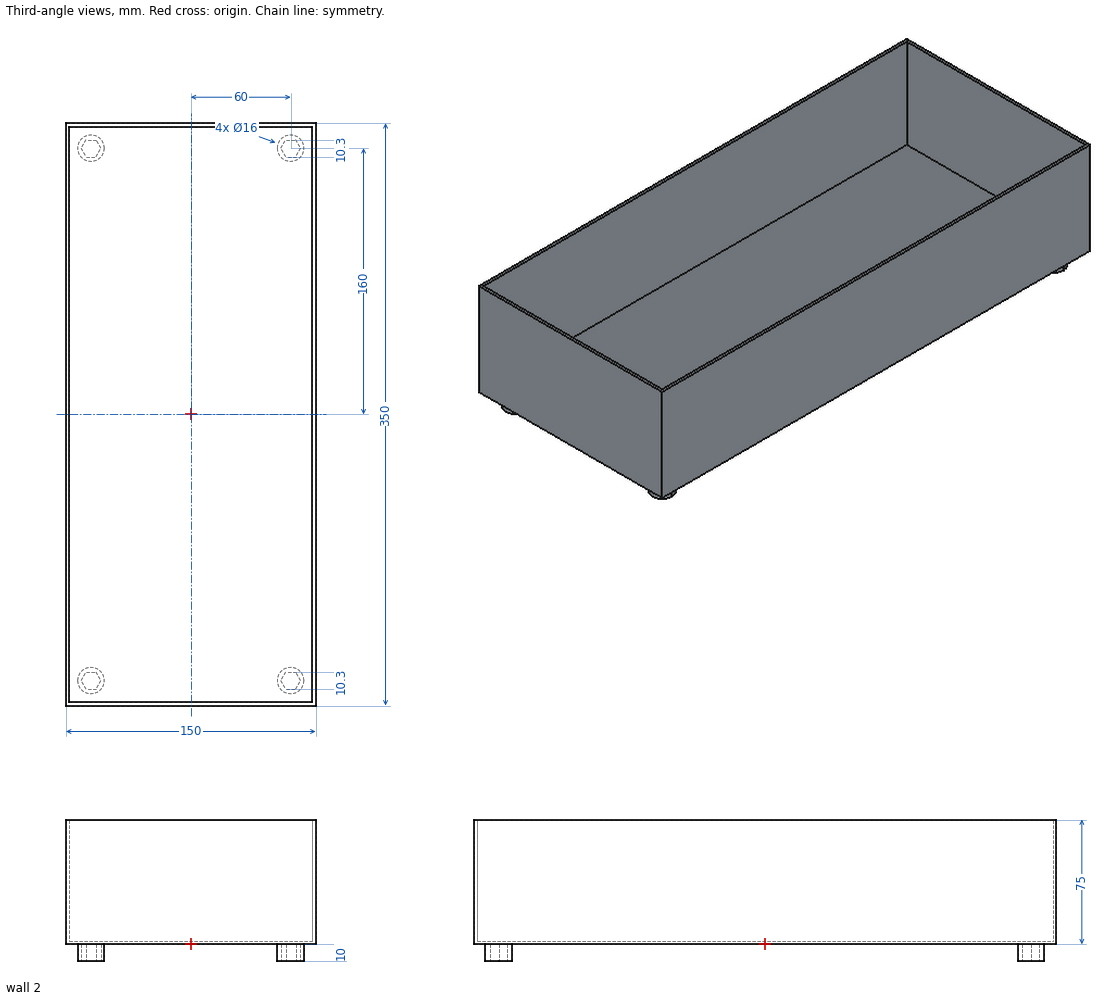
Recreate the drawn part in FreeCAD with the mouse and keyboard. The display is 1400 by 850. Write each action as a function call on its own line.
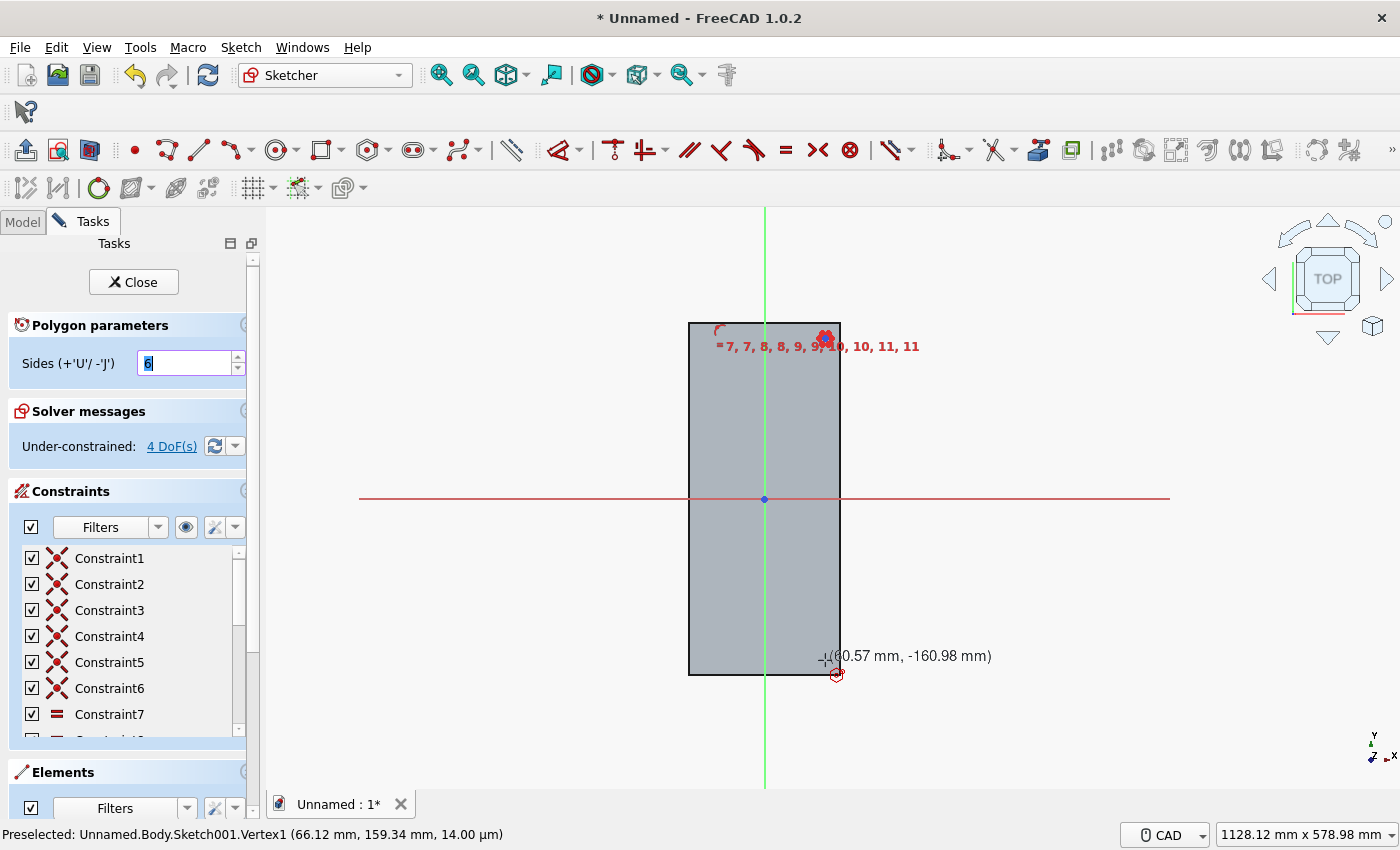
click(825, 660)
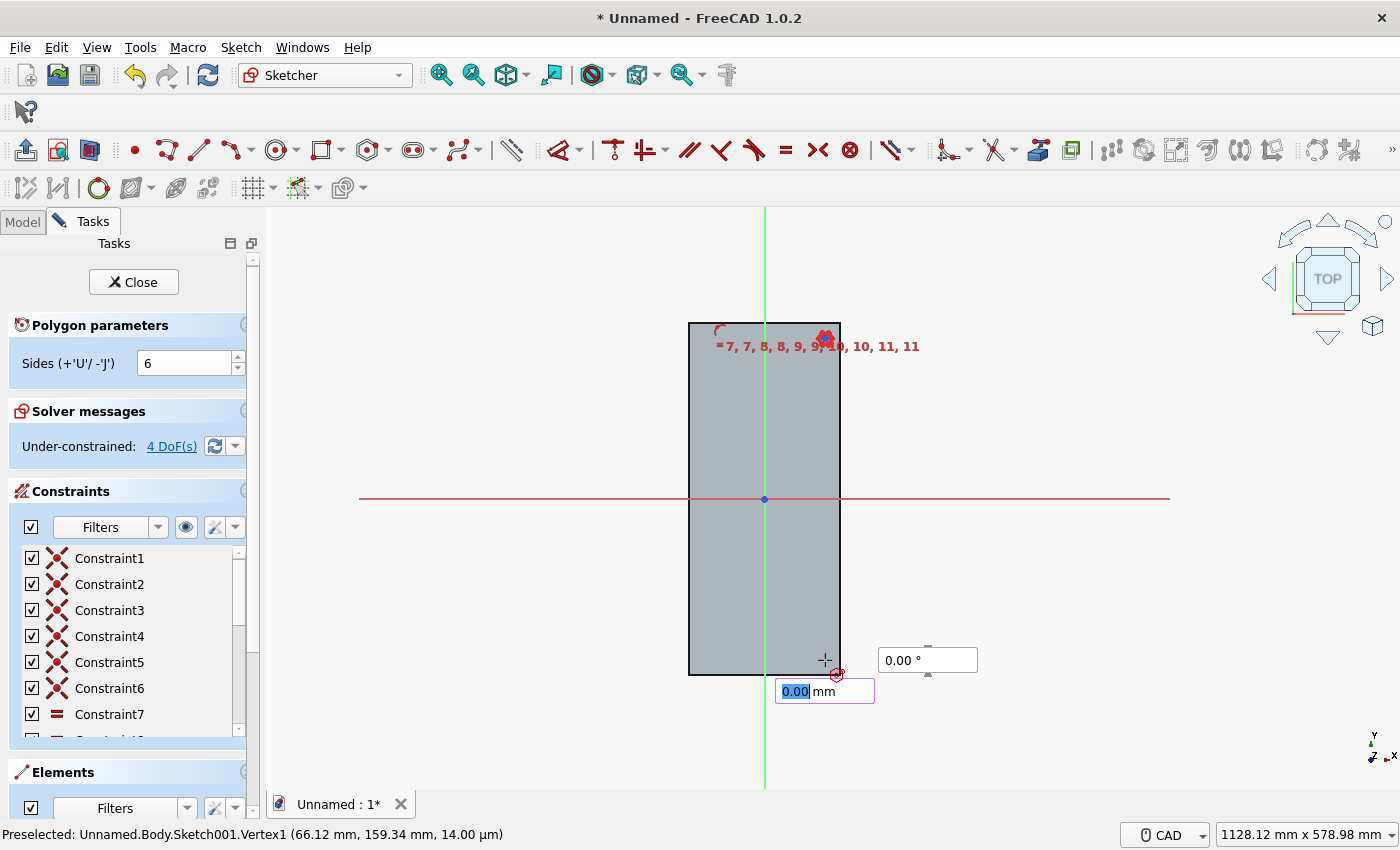
click(831, 660)
key(Escape)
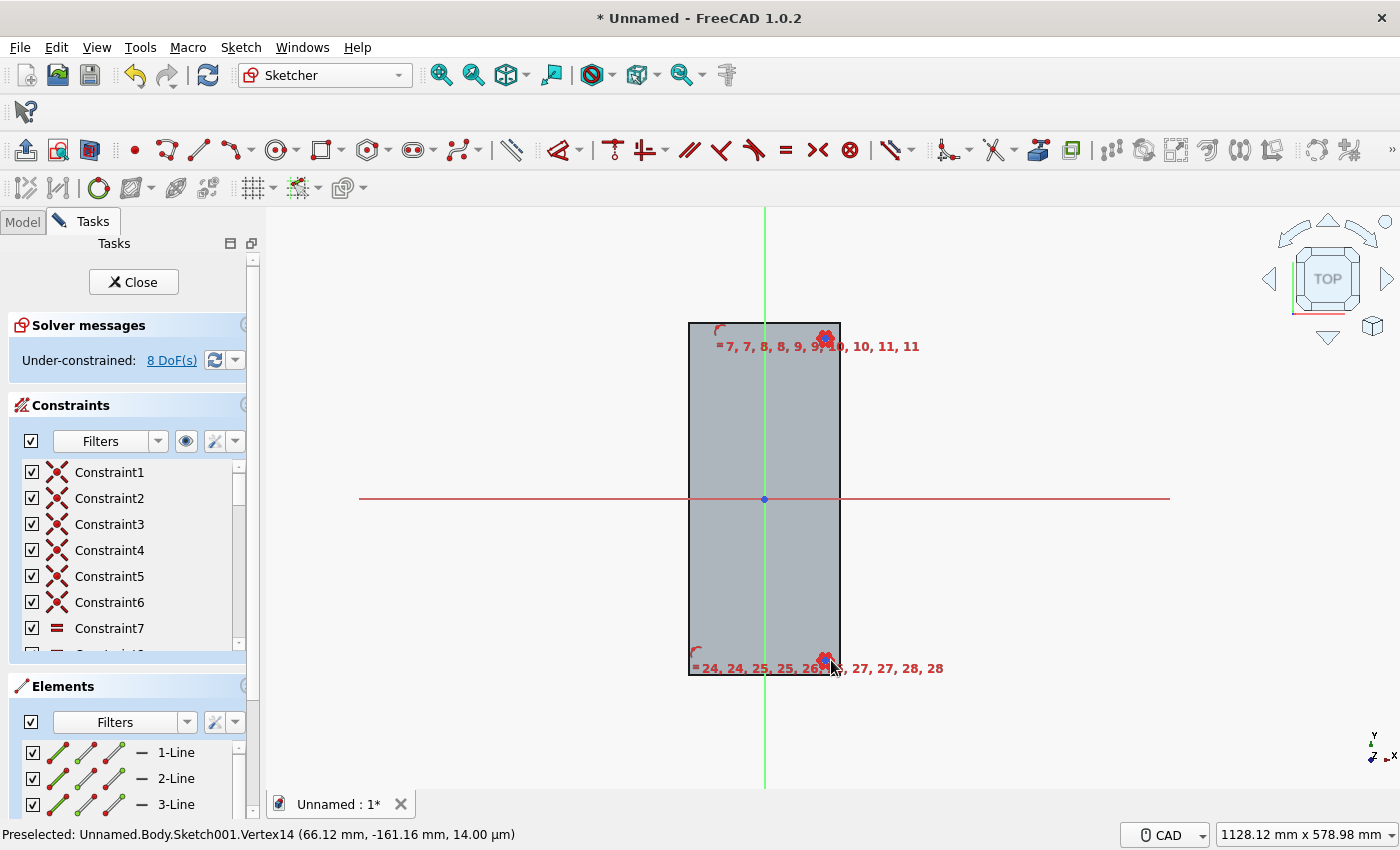
click(368, 150)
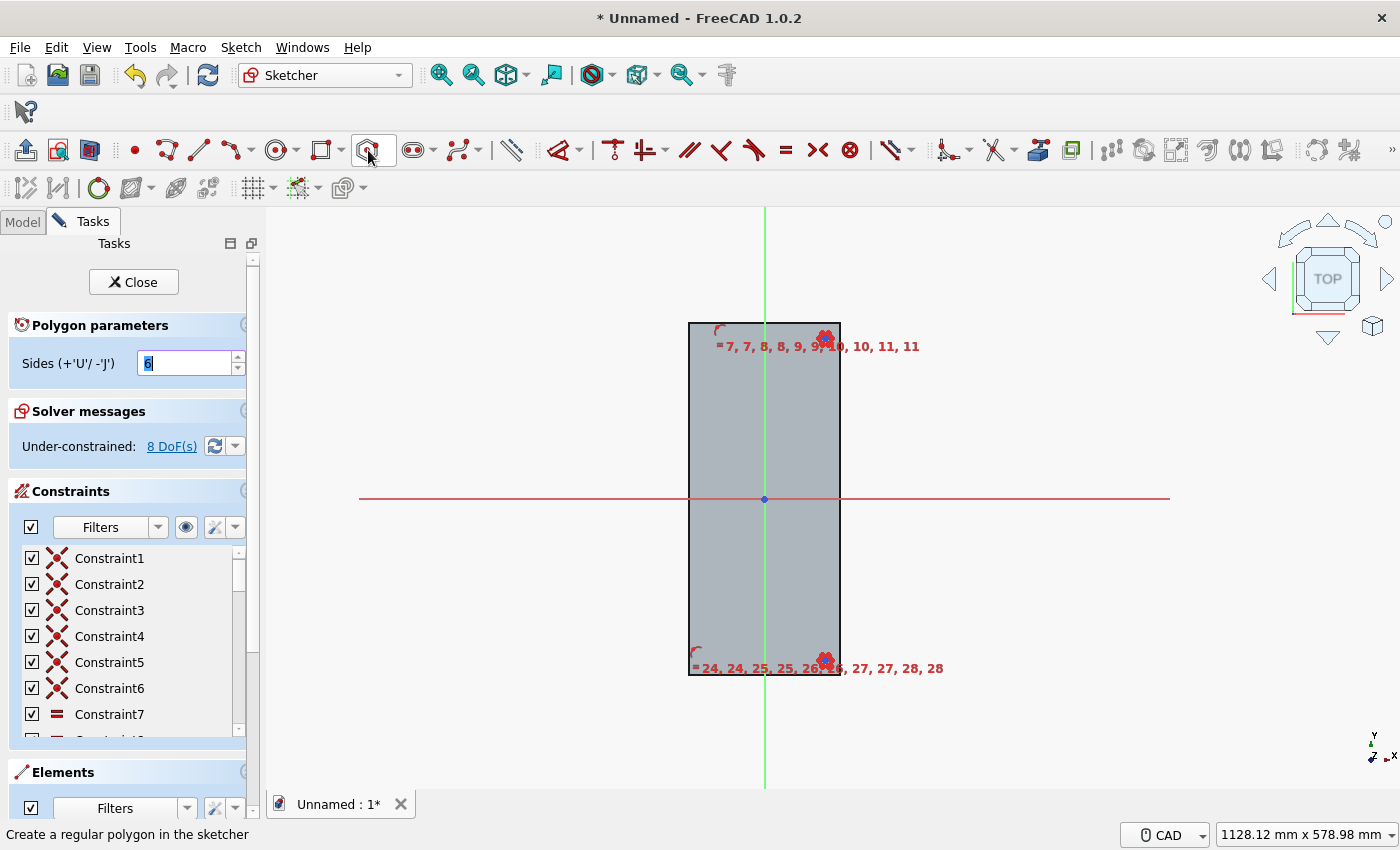
scroll(704, 660, up, 9)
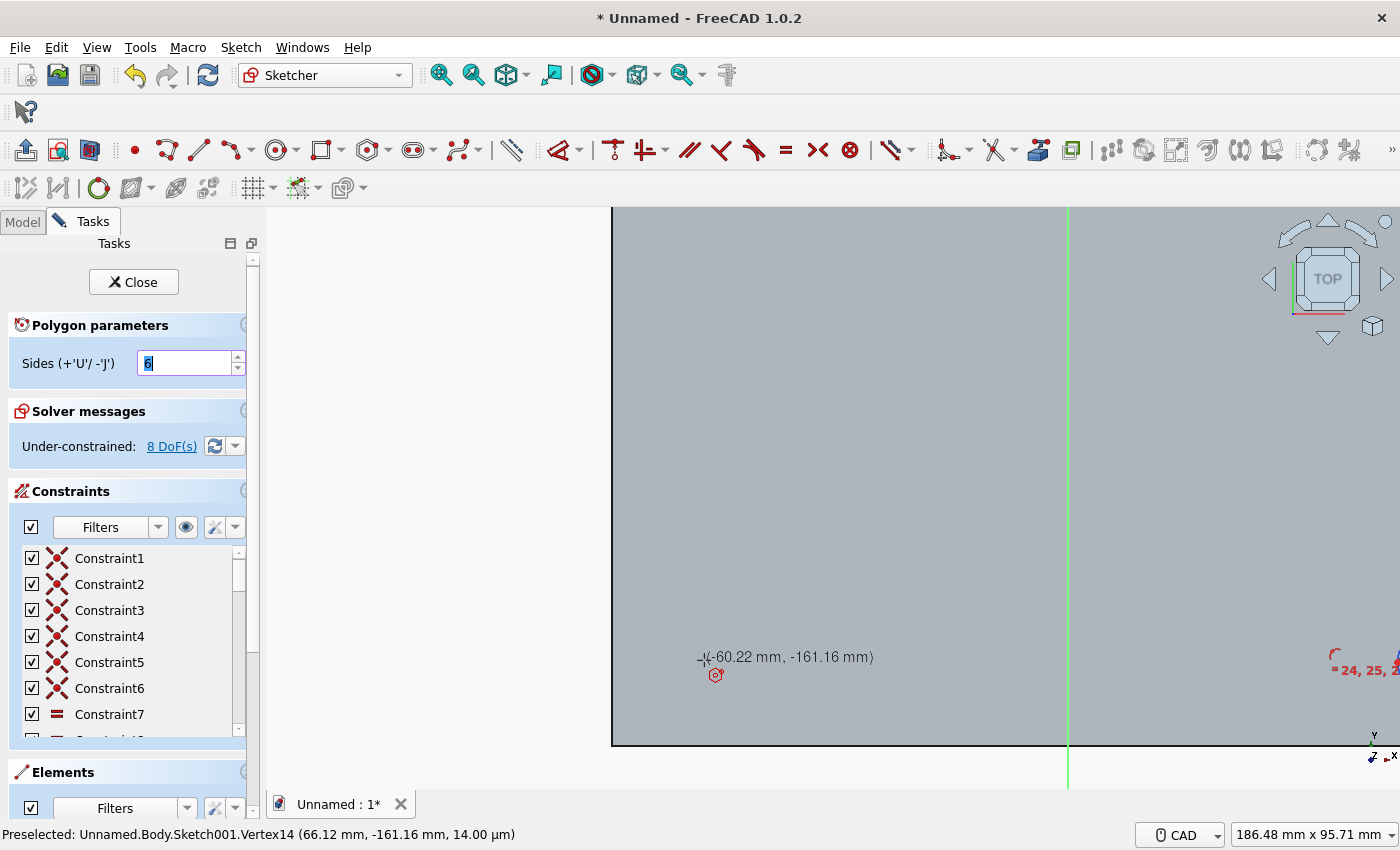
scroll(704, 660, down, 9)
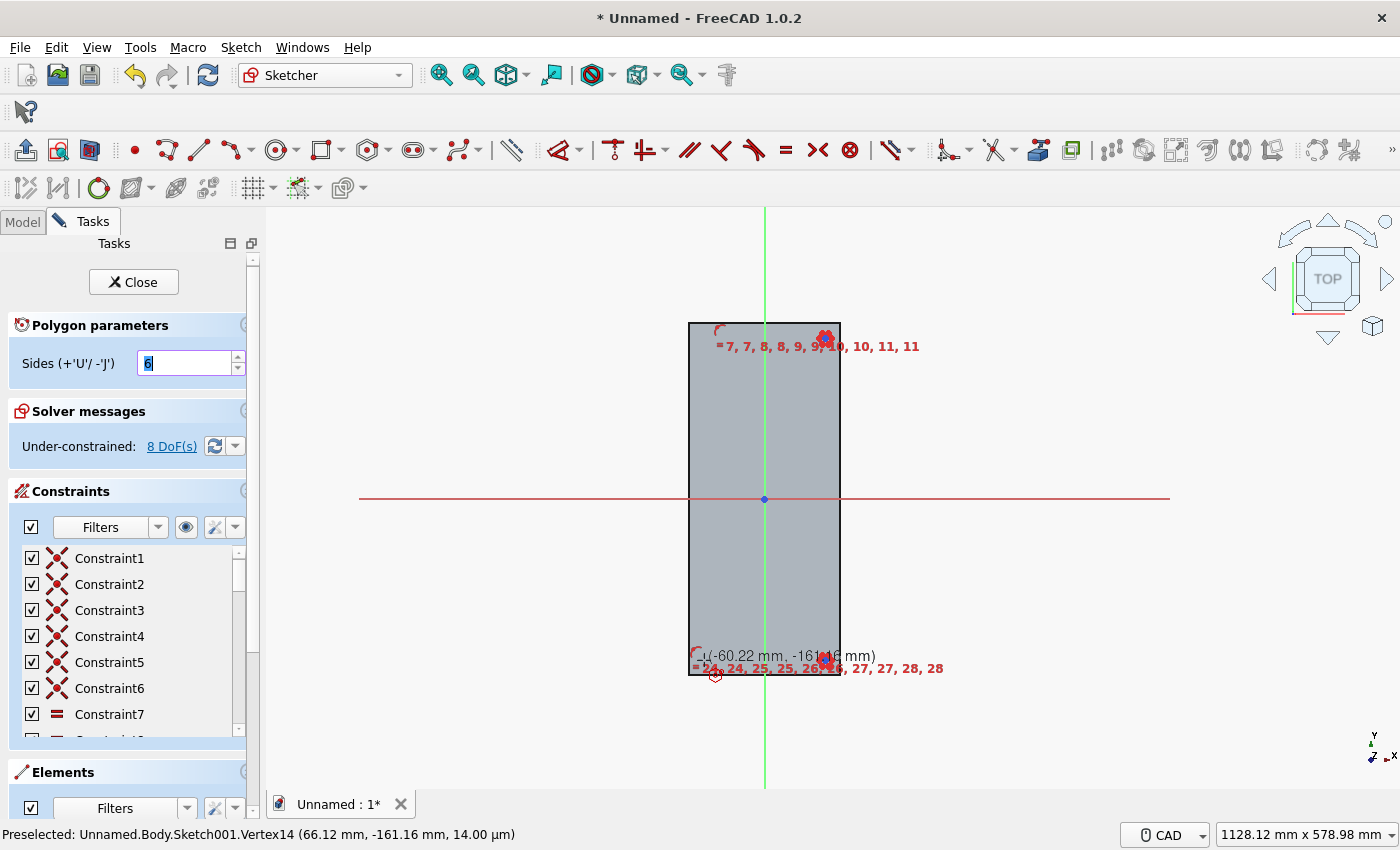
click(704, 660)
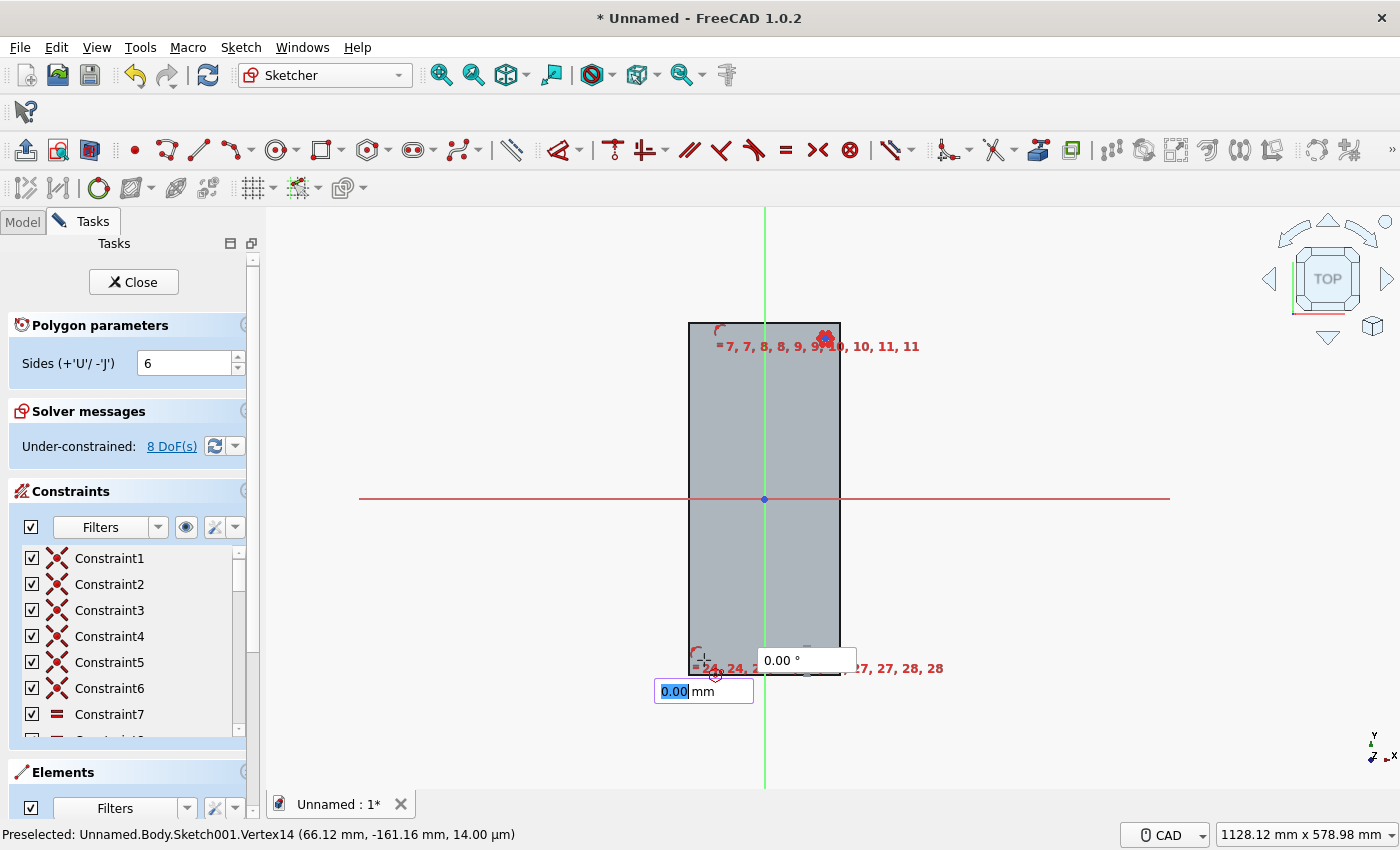
click(698, 660)
key(Escape)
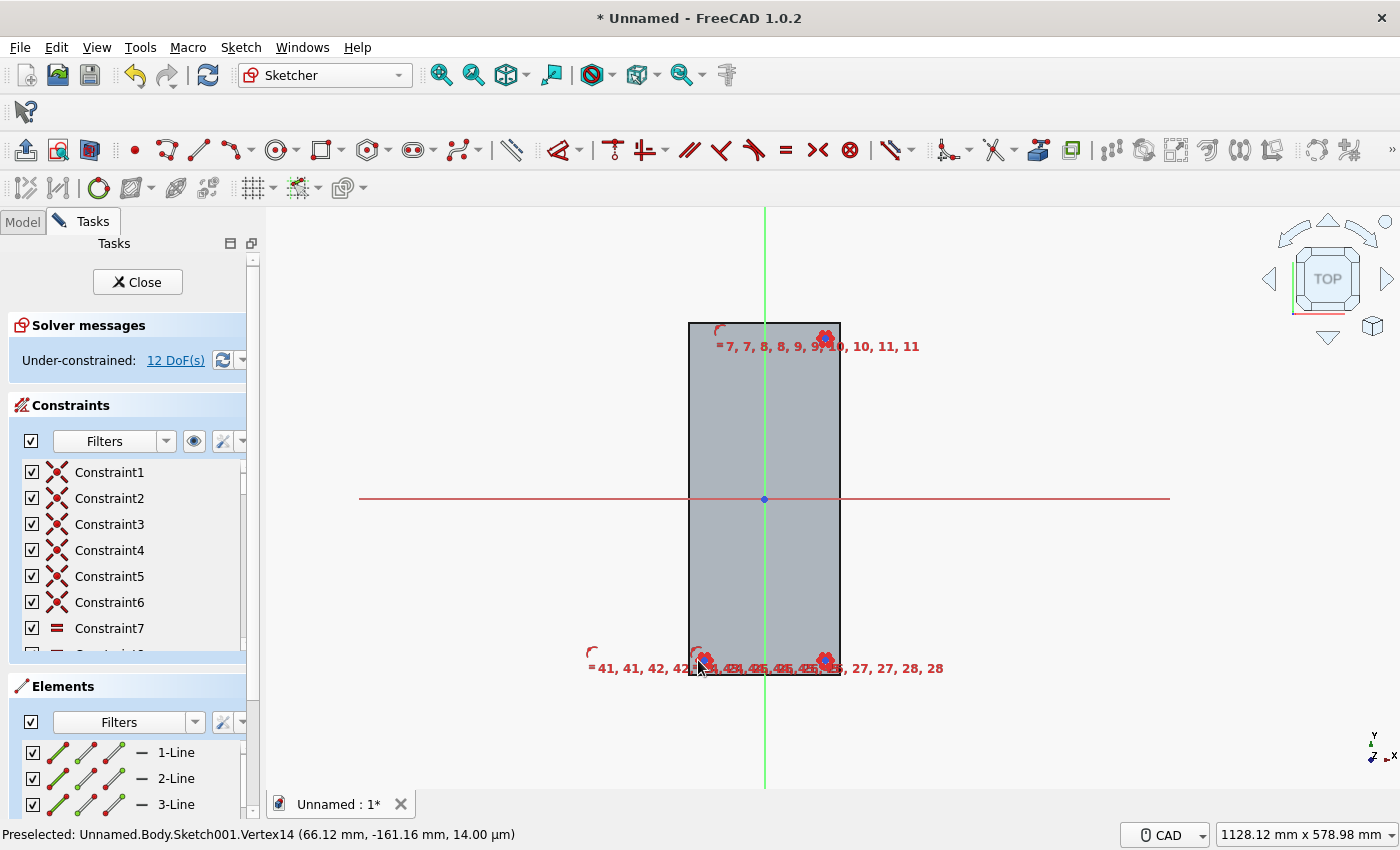
click(368, 150)